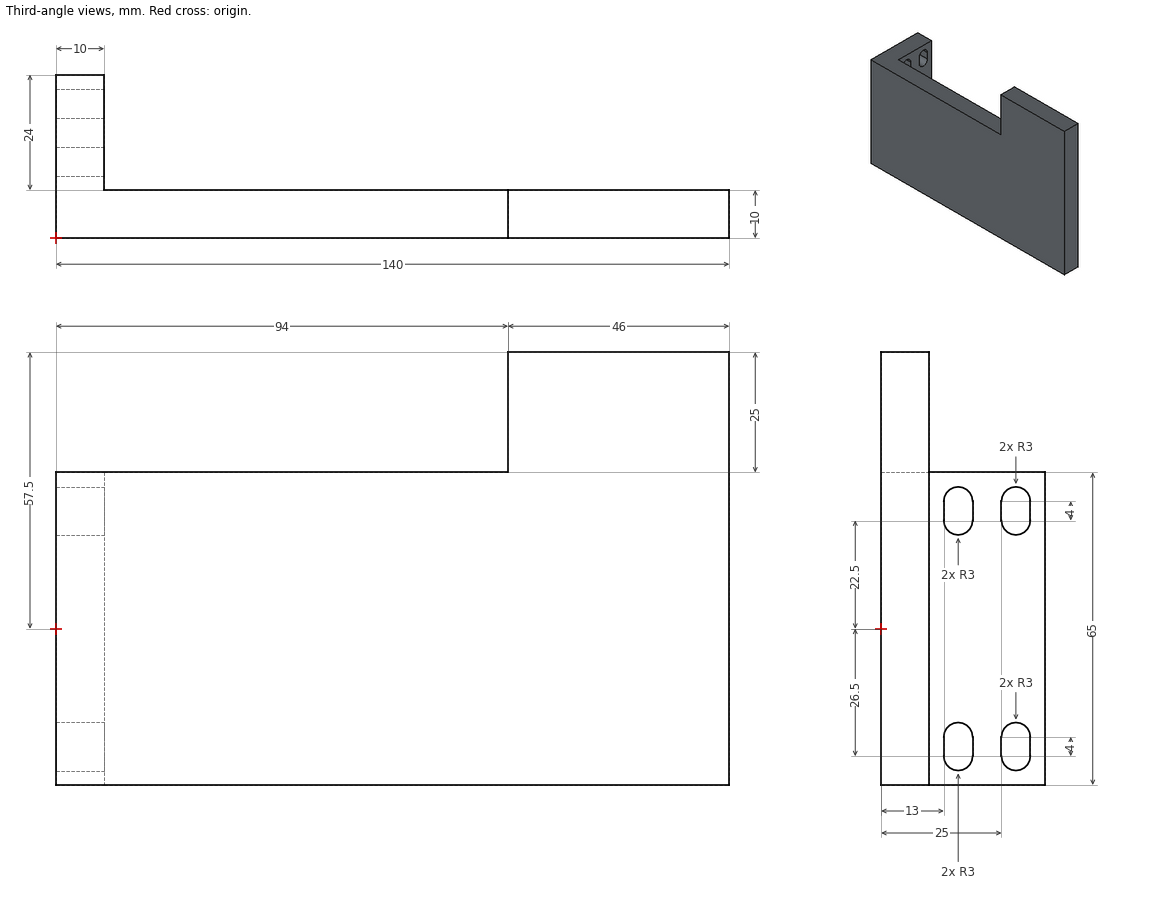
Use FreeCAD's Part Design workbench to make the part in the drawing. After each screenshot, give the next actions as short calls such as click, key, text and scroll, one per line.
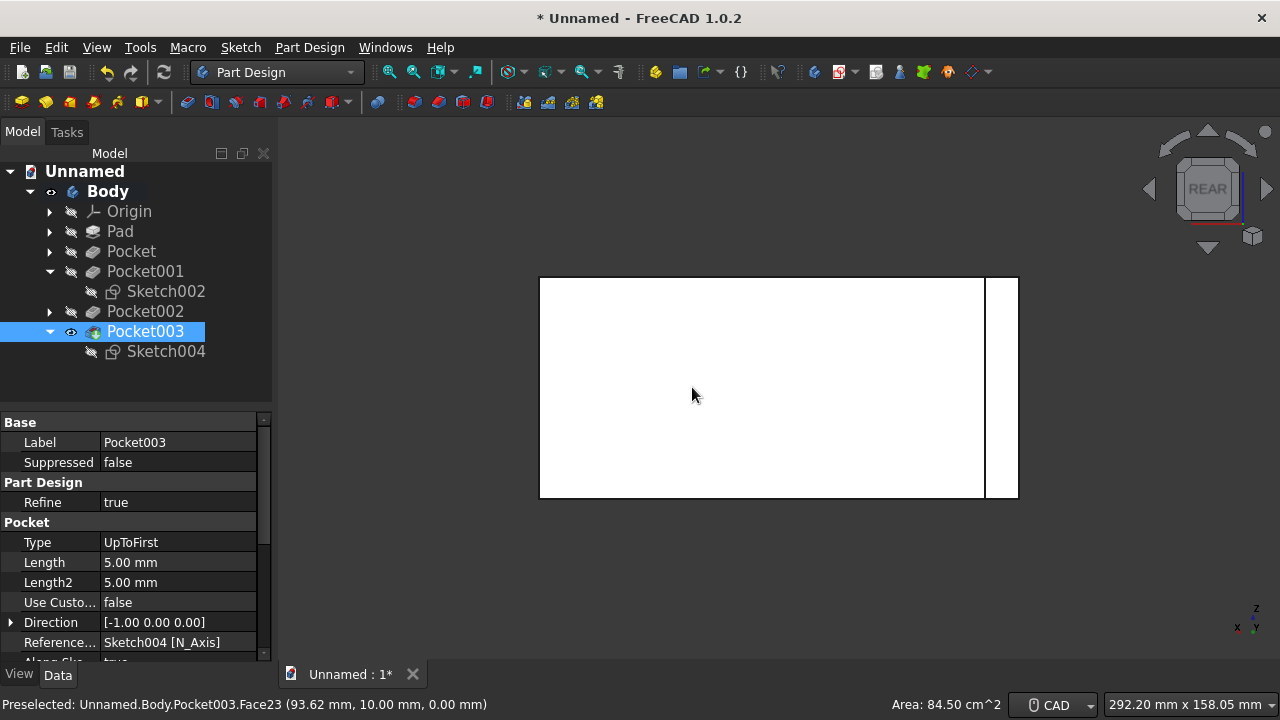
click(840, 72)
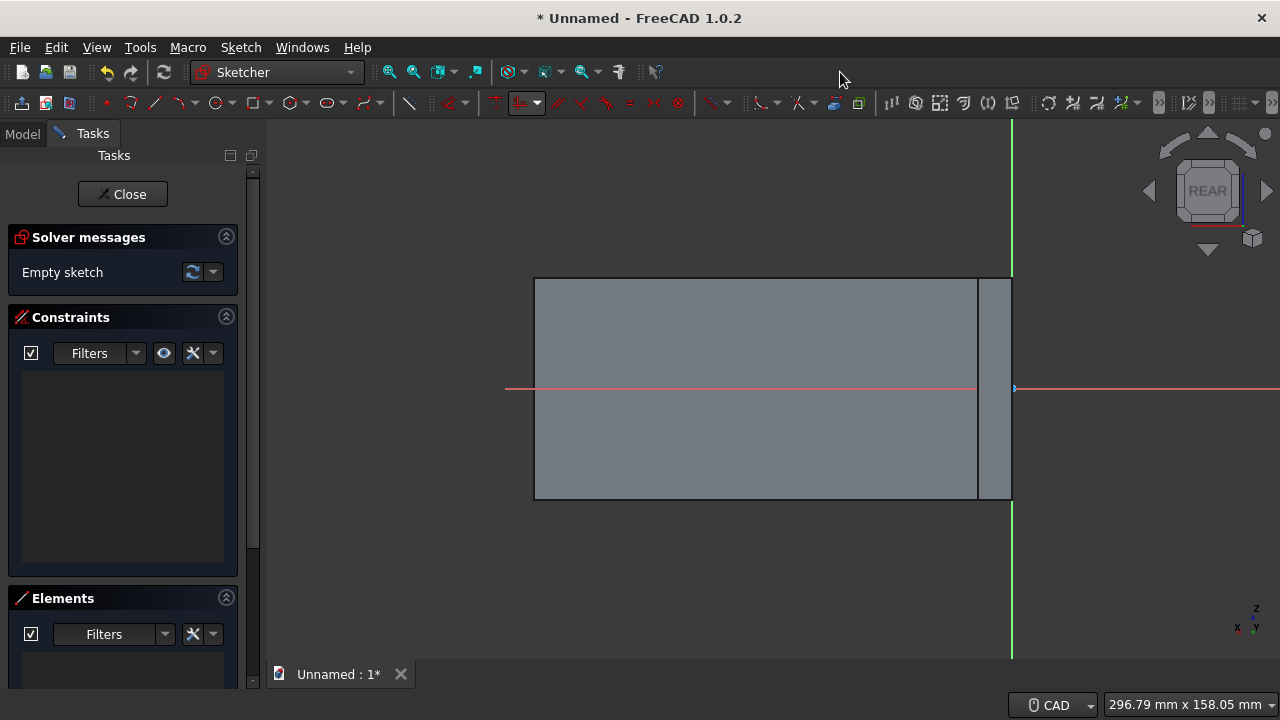
scroll(582, 185, up, 7)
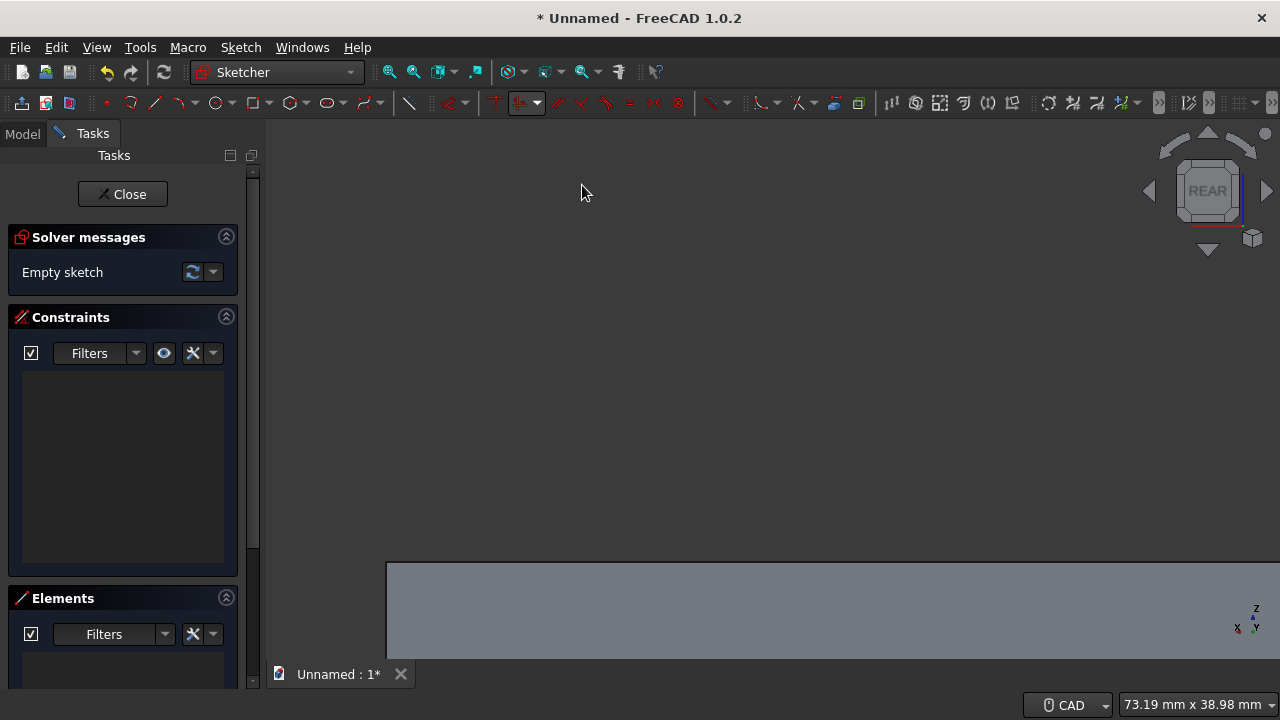
click(254, 104)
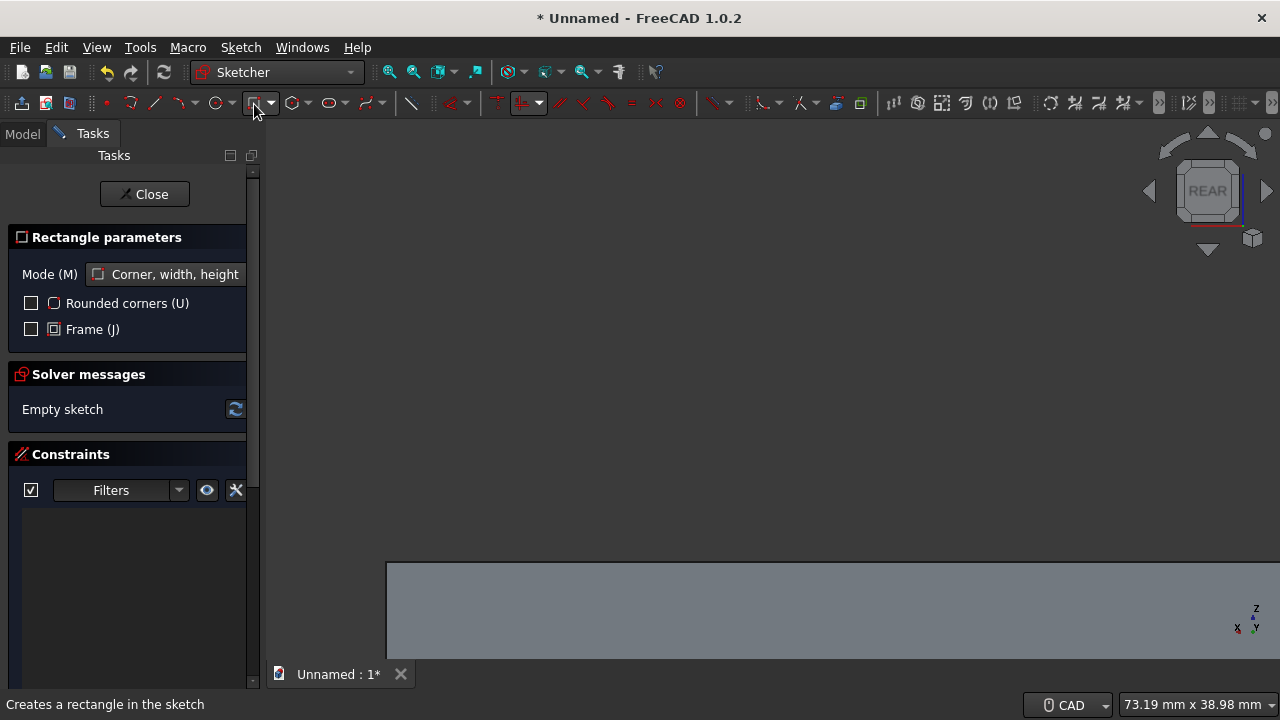
click(386, 215)
move(1023, 562)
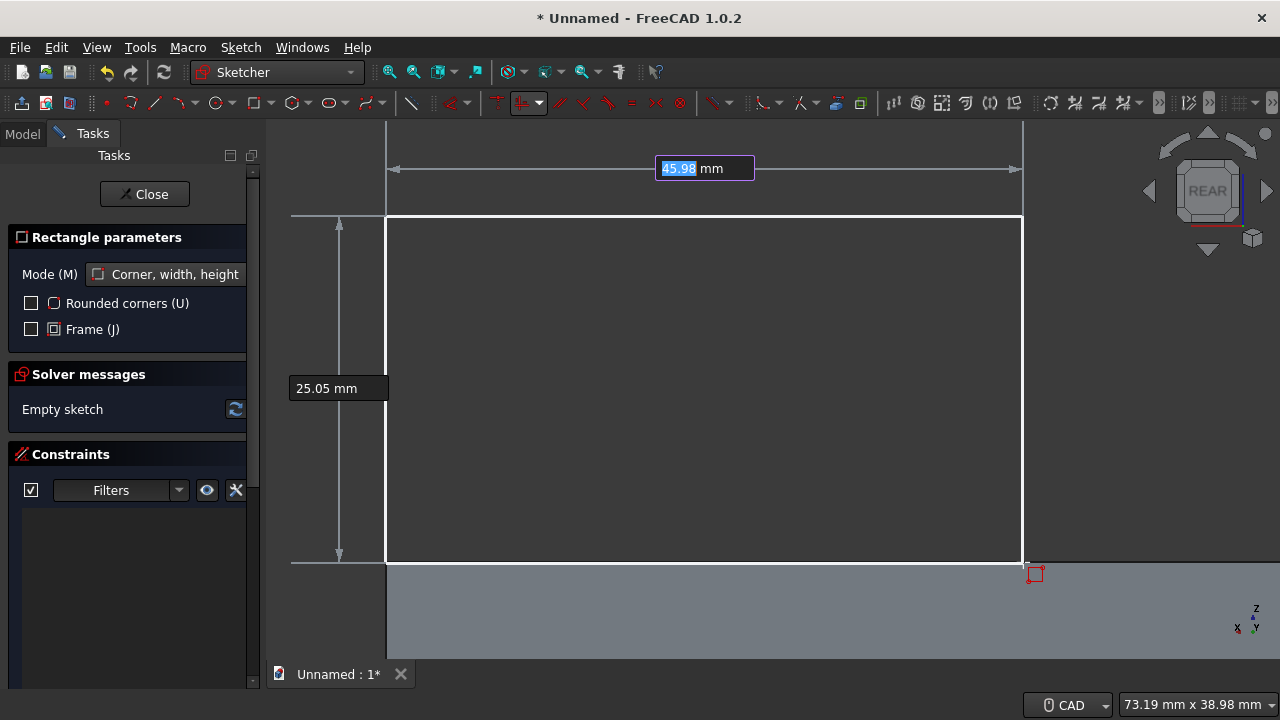
text(46)
key(Tab)
text(25)
key(Return)
key(Escape)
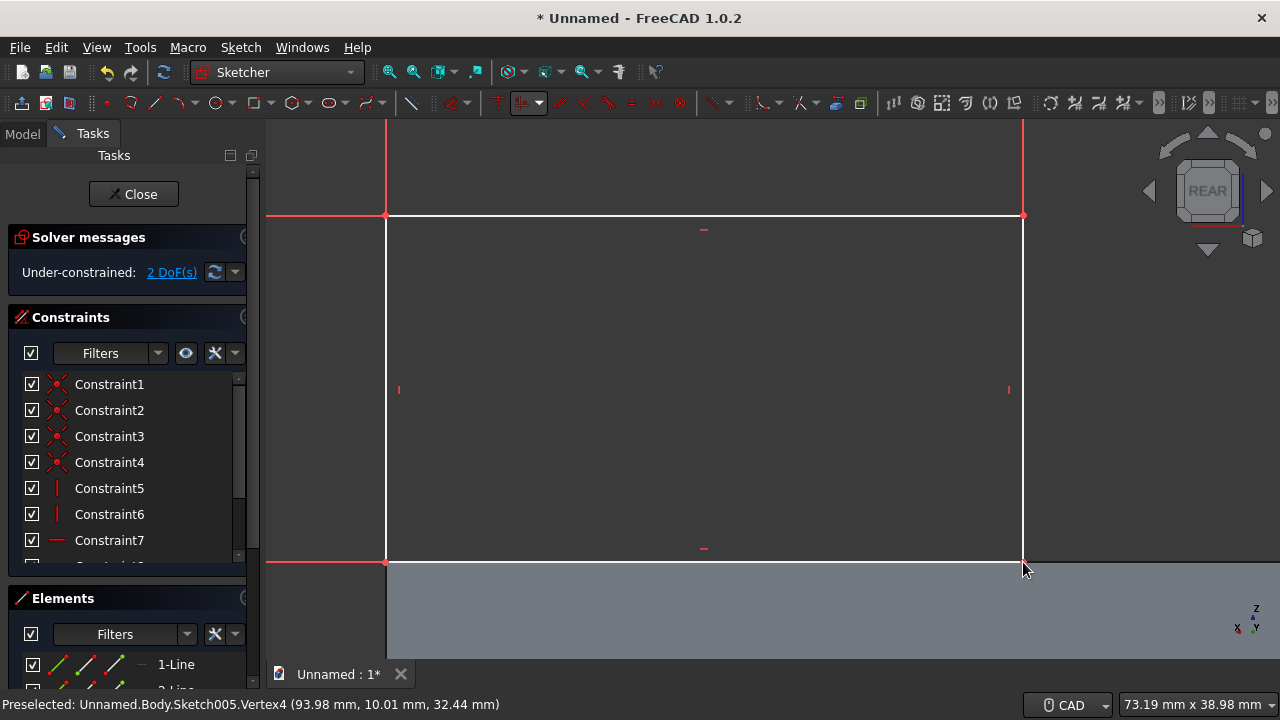
click(450, 104)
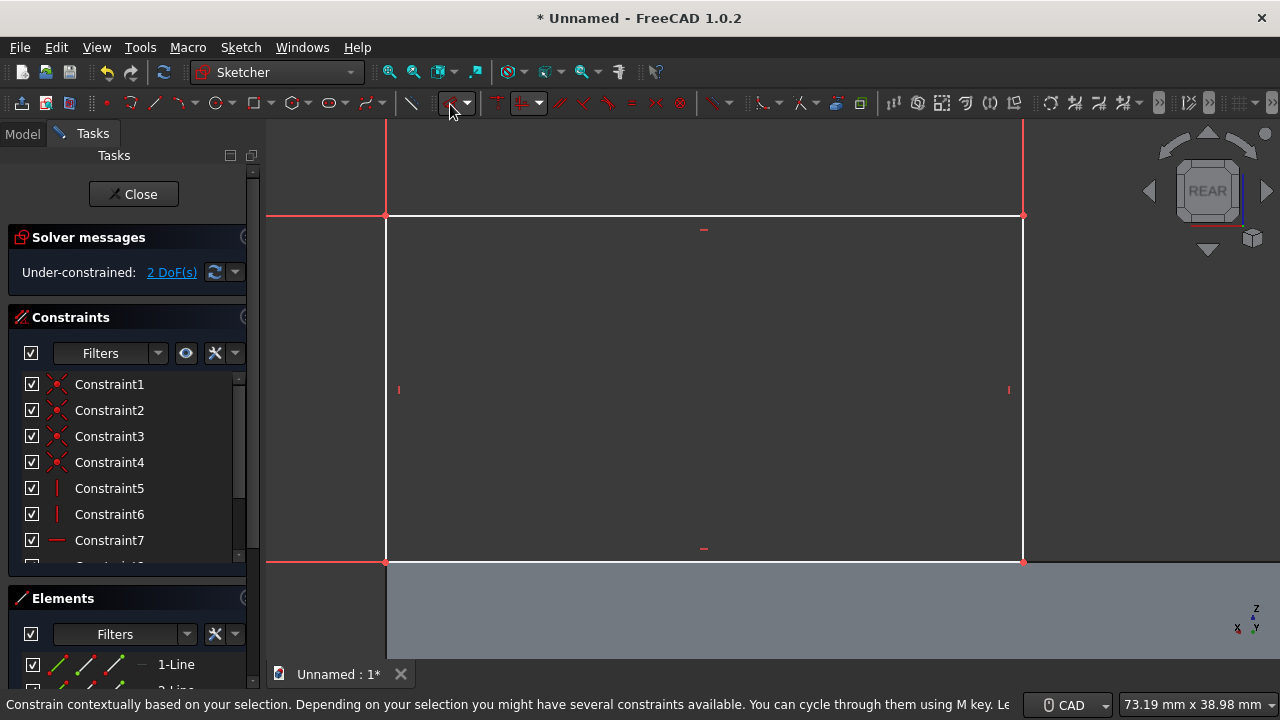
click(1023, 562)
click(1069, 528)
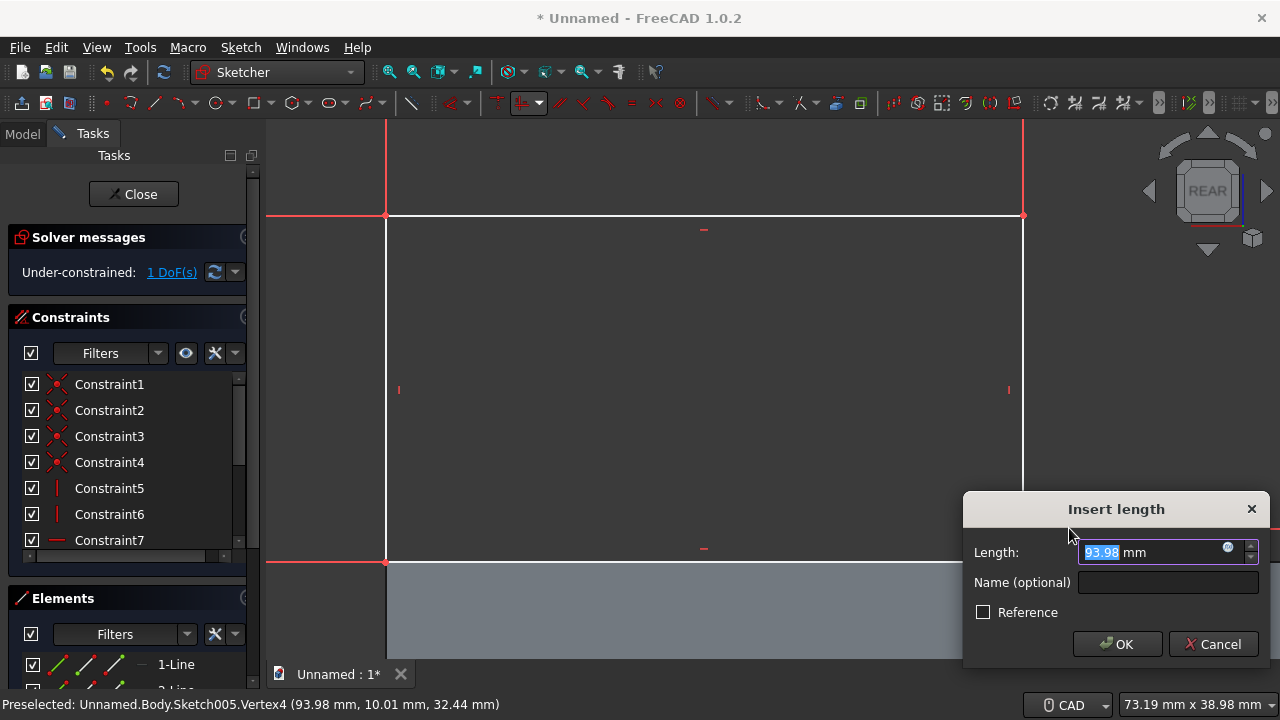
text(94)
key(Return)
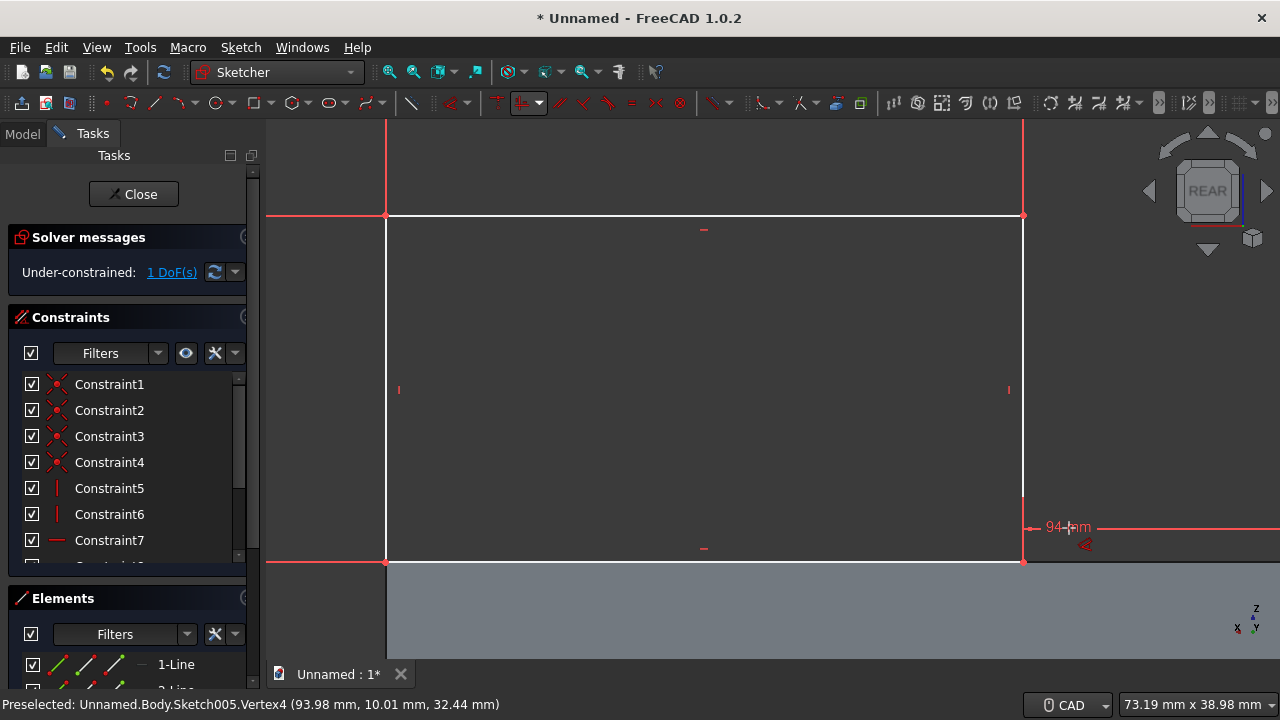
click(386, 216)
click(352, 424)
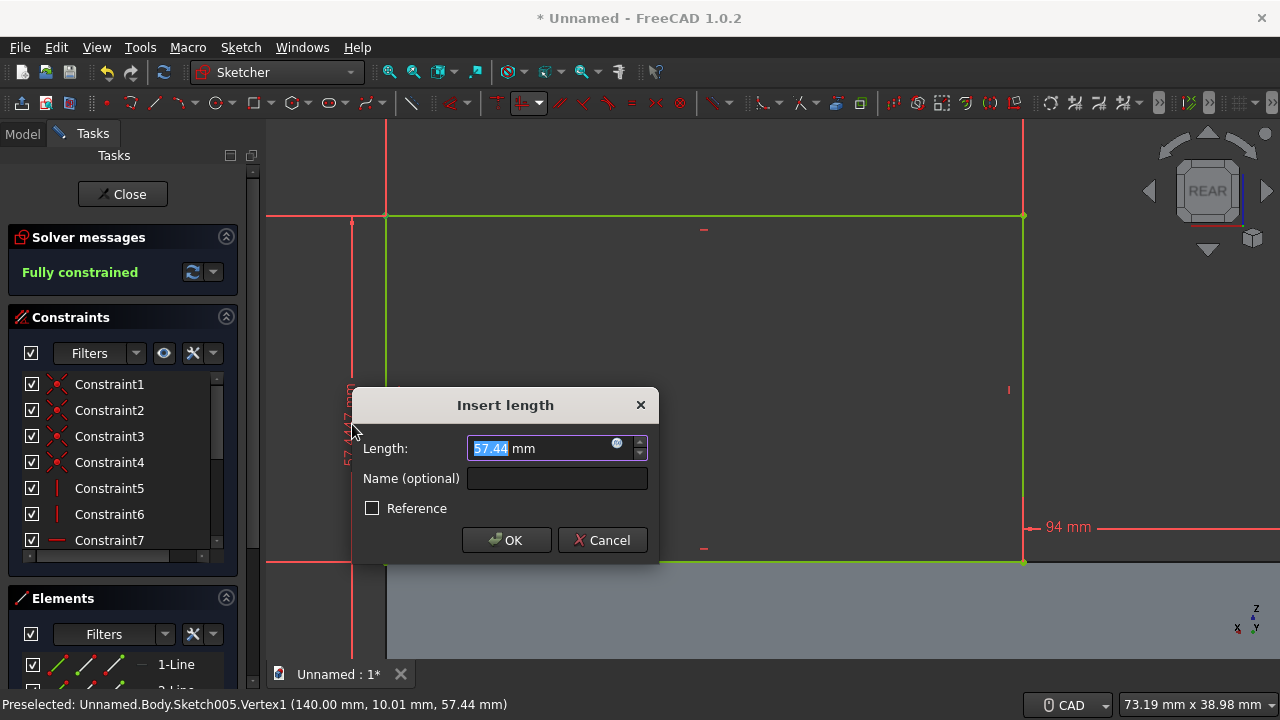
text(57.5)
key(Return)
key(Escape)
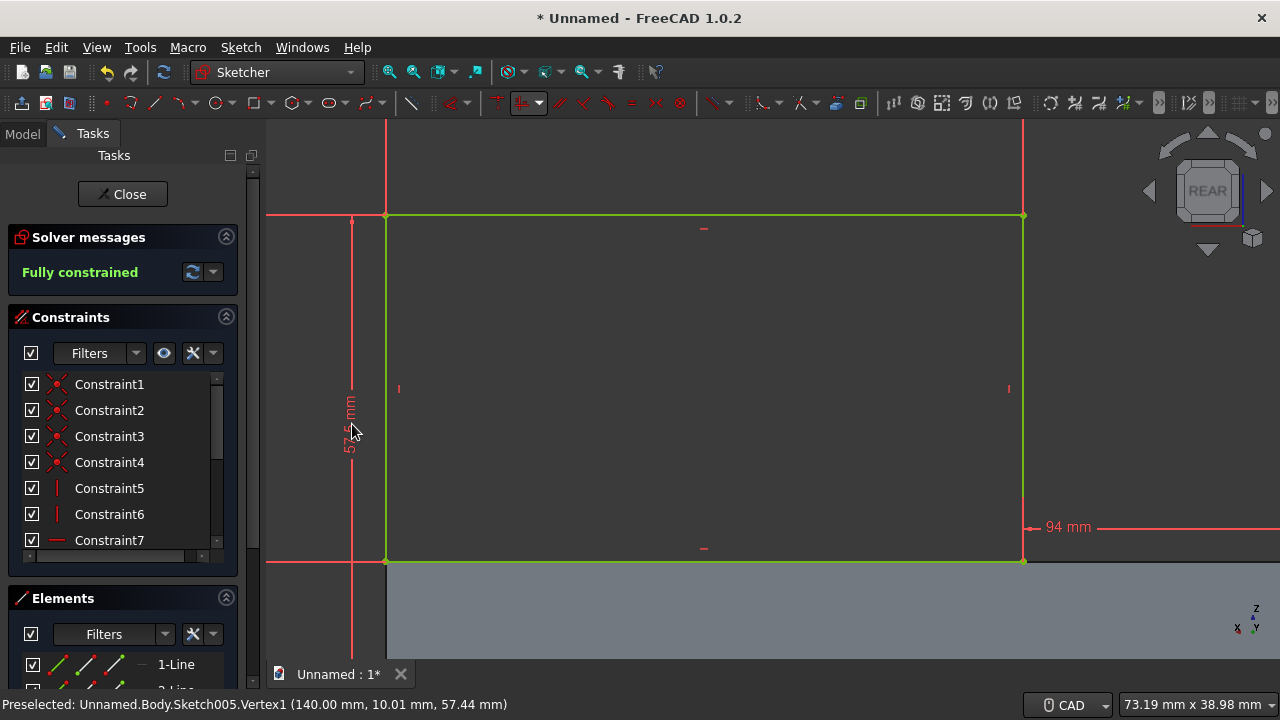
click(123, 194)